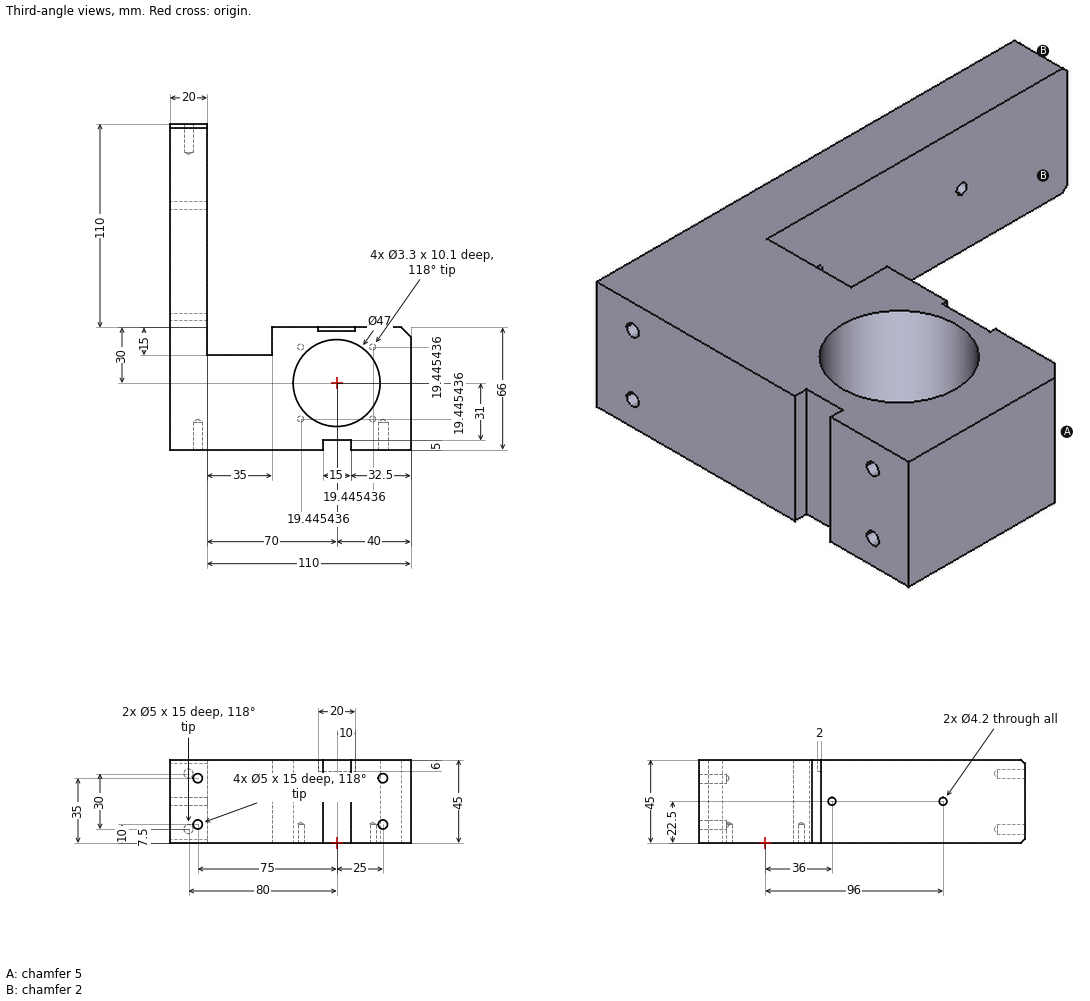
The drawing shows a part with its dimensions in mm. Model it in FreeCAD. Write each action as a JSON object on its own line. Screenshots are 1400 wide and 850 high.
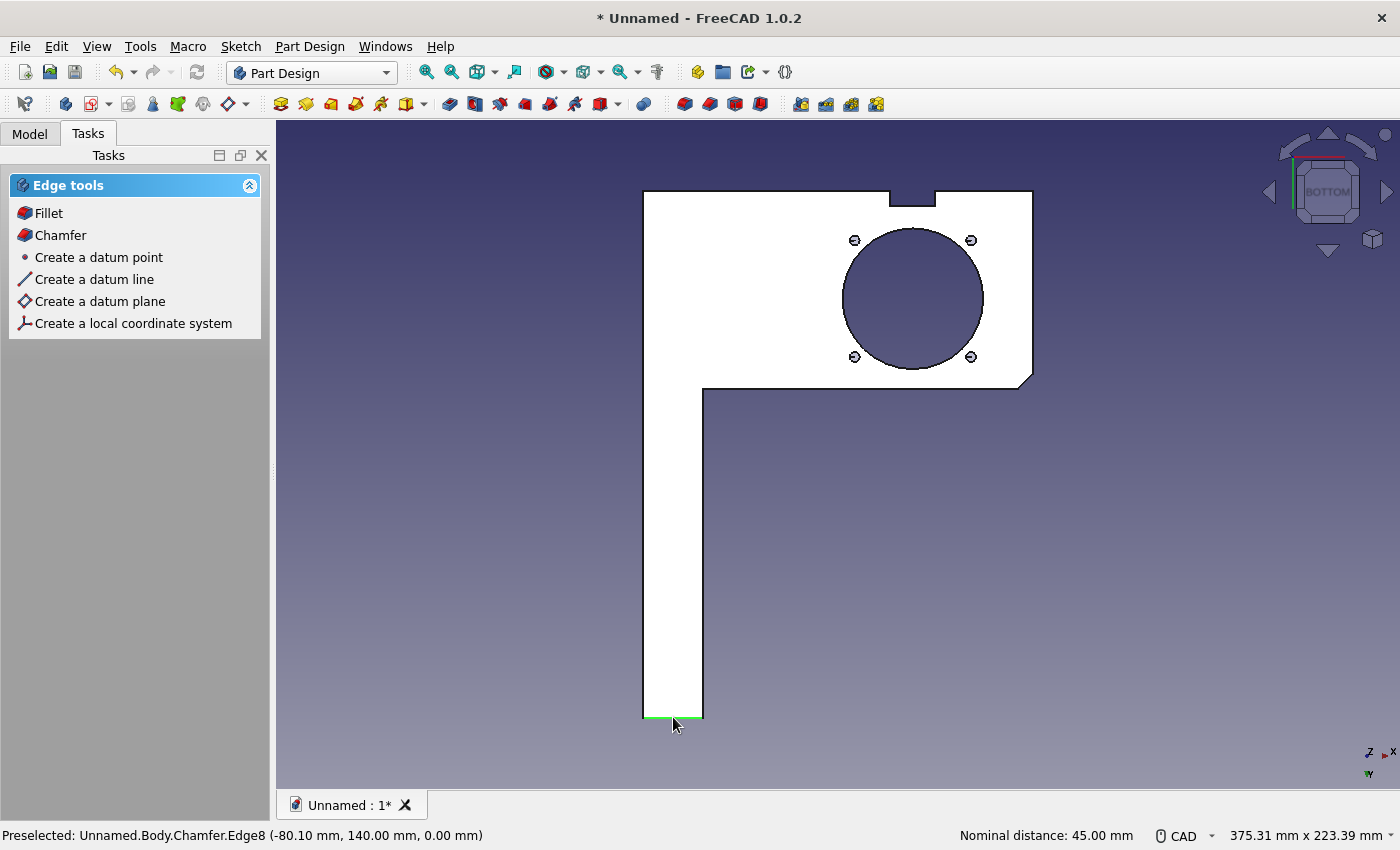
{"action": "left_click", "coordinate": [710, 104]}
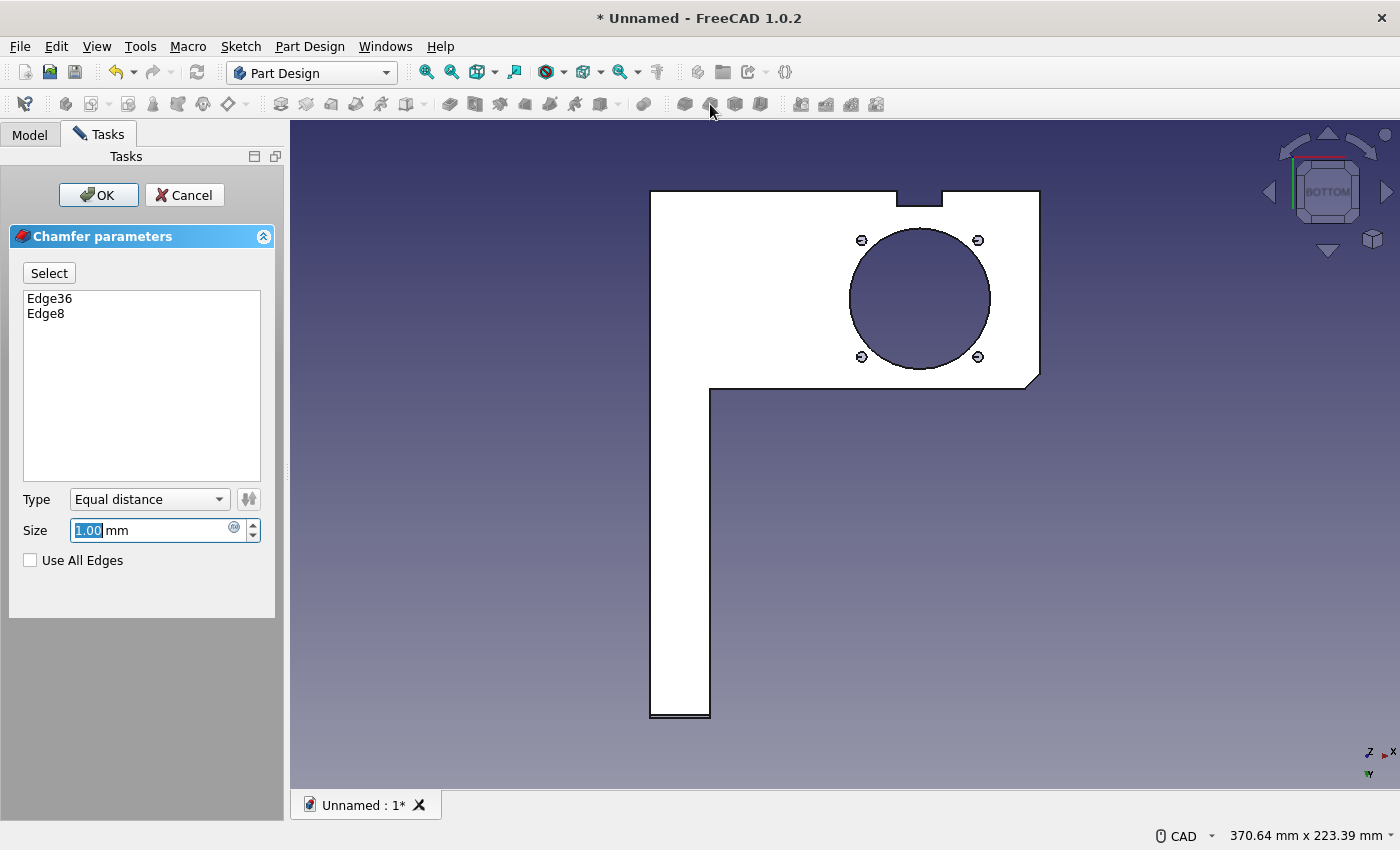
{"action": "type", "text": "2"}
{"action": "key", "text": "Tab"}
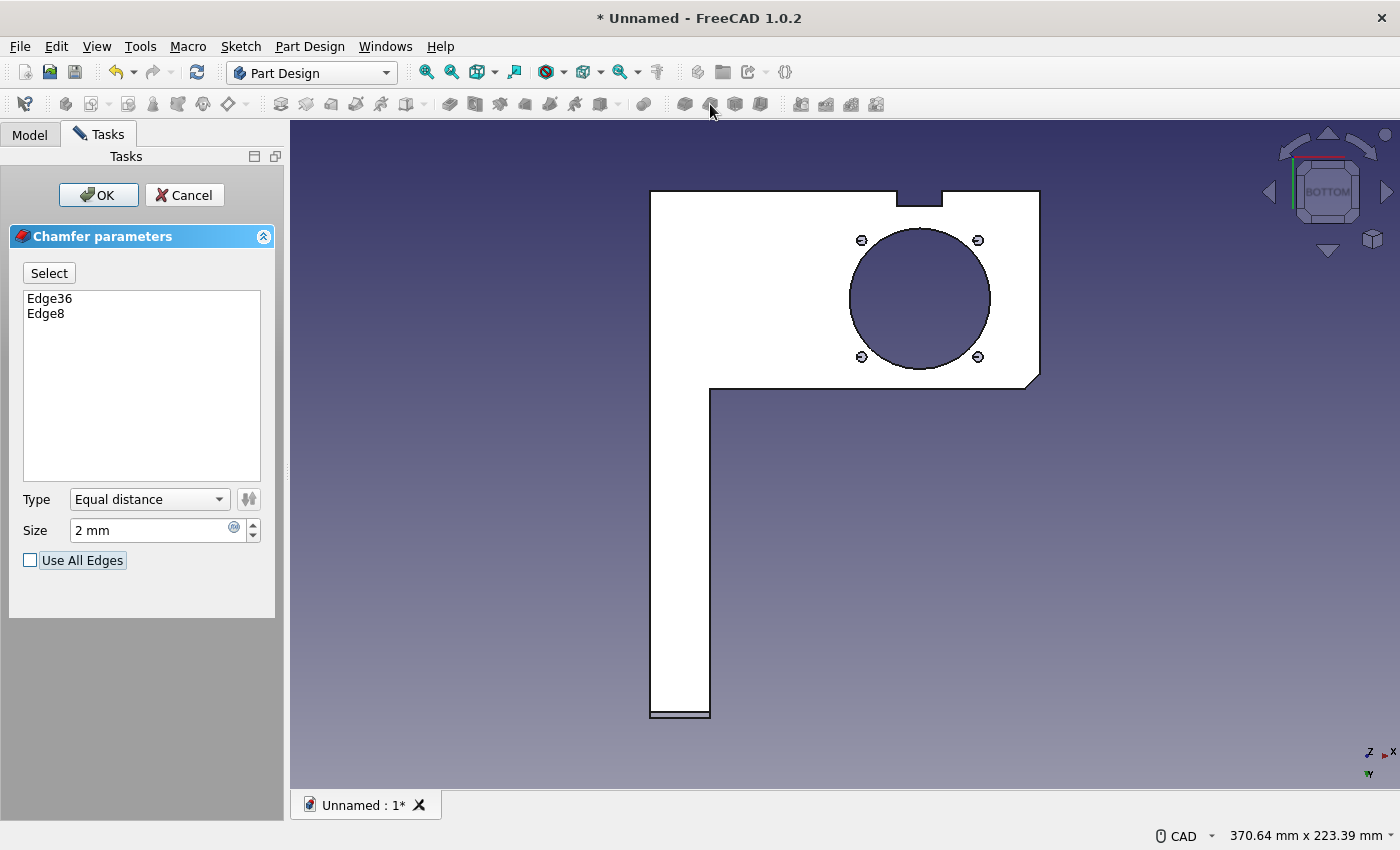
{"action": "left_click", "coordinate": [99, 195]}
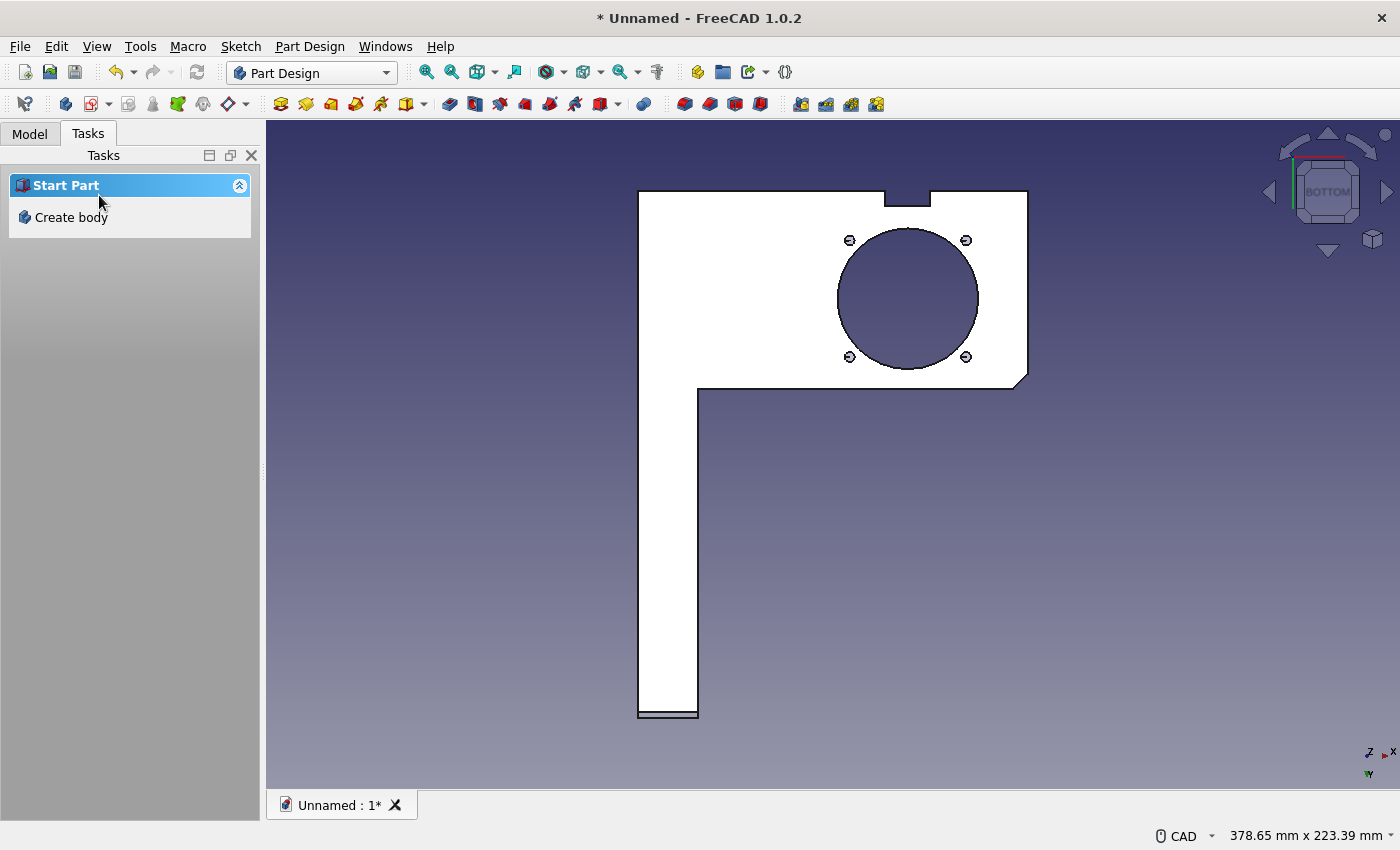
{"action": "left_click", "coordinate": [90, 104]}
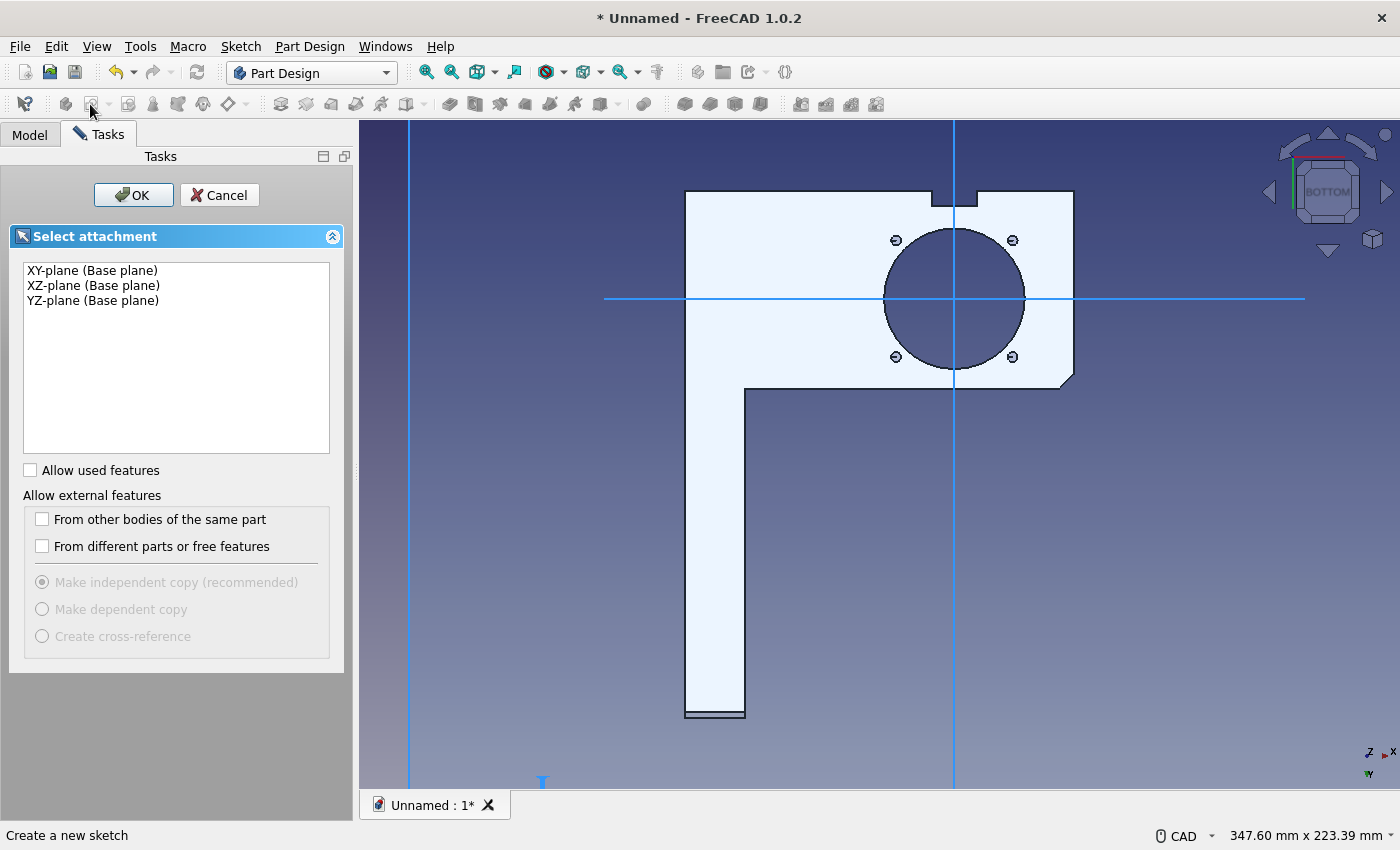
{"action": "left_click", "coordinate": [84, 270]}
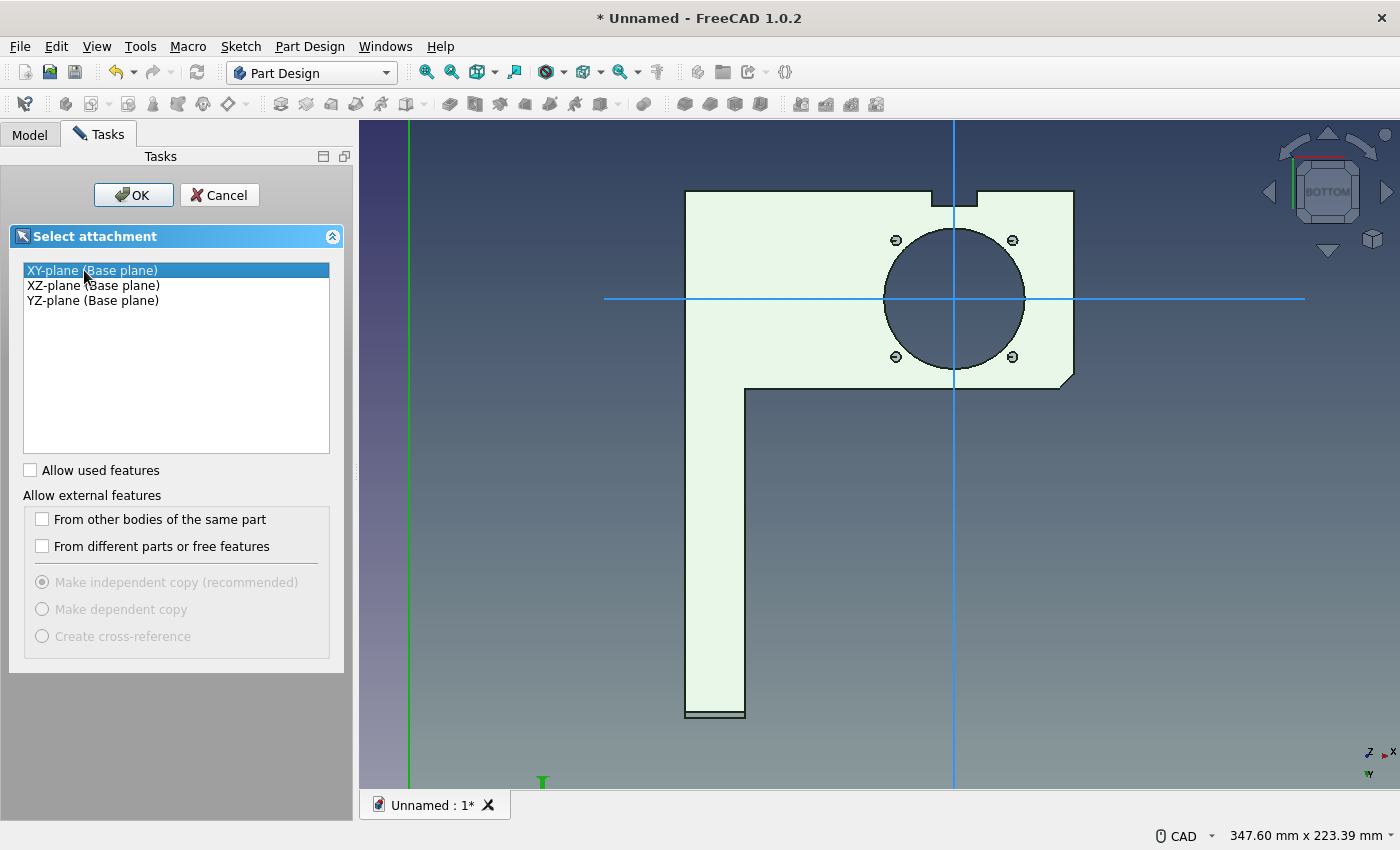
{"action": "left_click", "coordinate": [134, 195]}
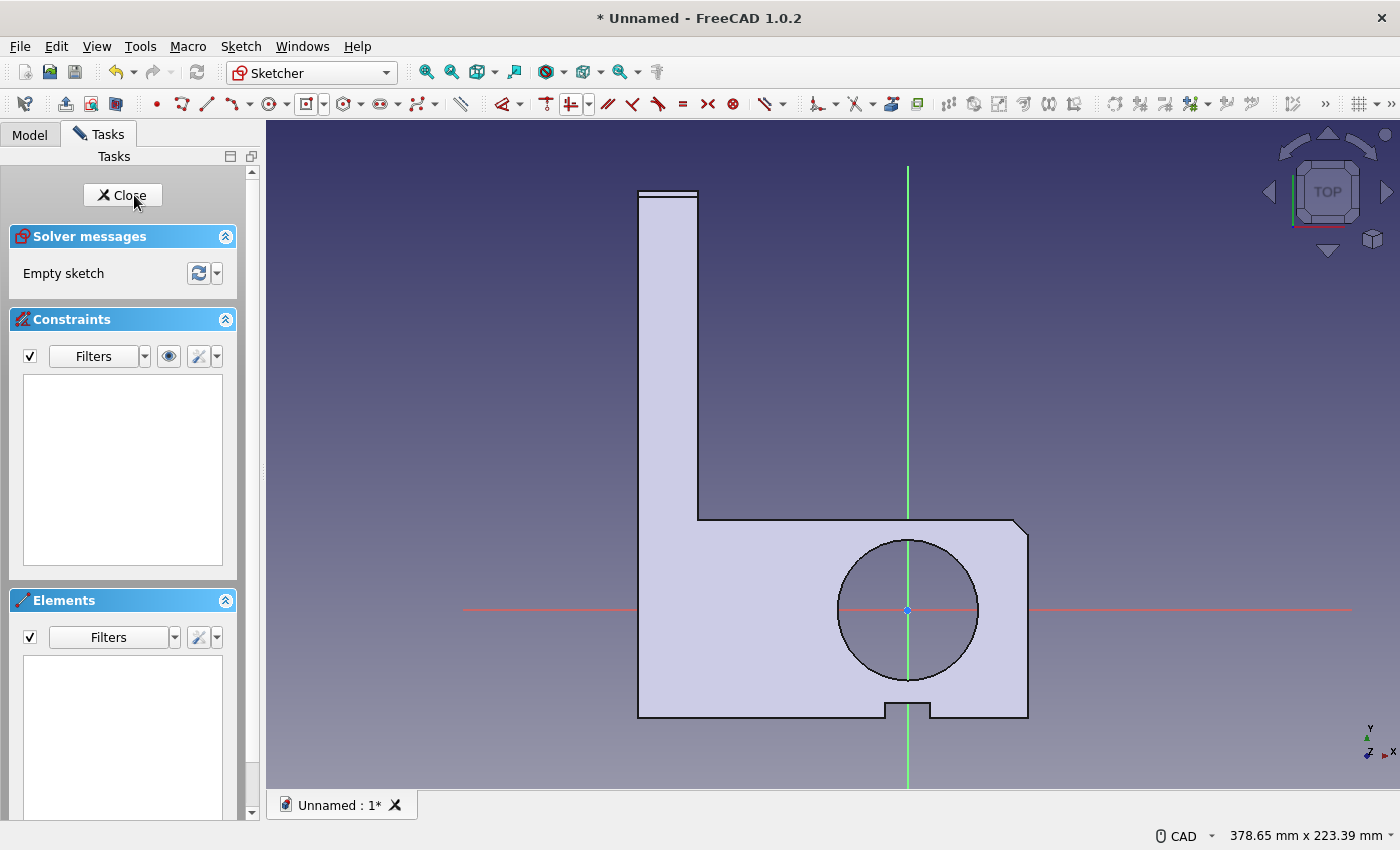
{"action": "key", "text": "q s"}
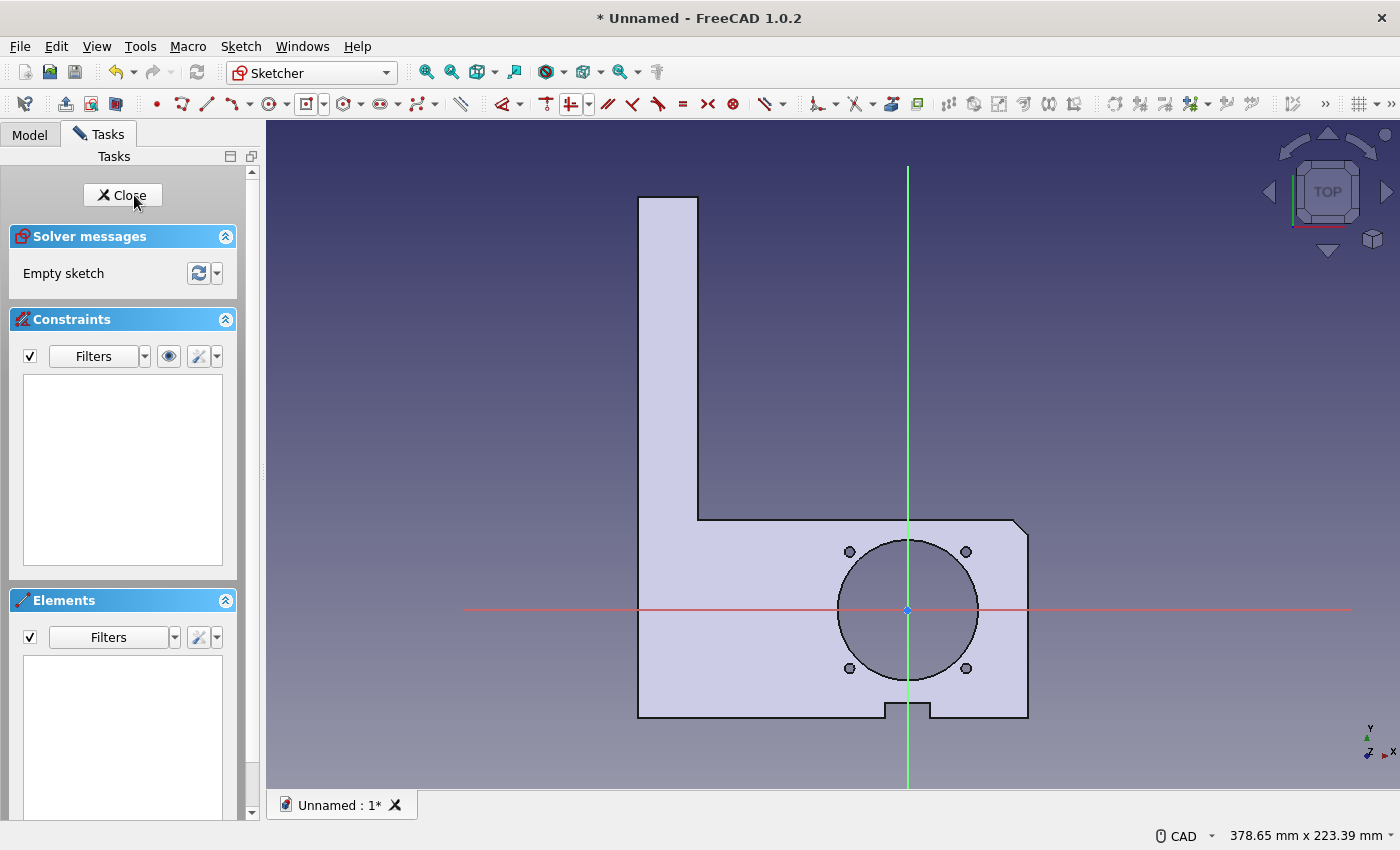
{"action": "scroll", "coordinate": [820, 613], "scroll_direction": "up", "scroll_amount": 6}